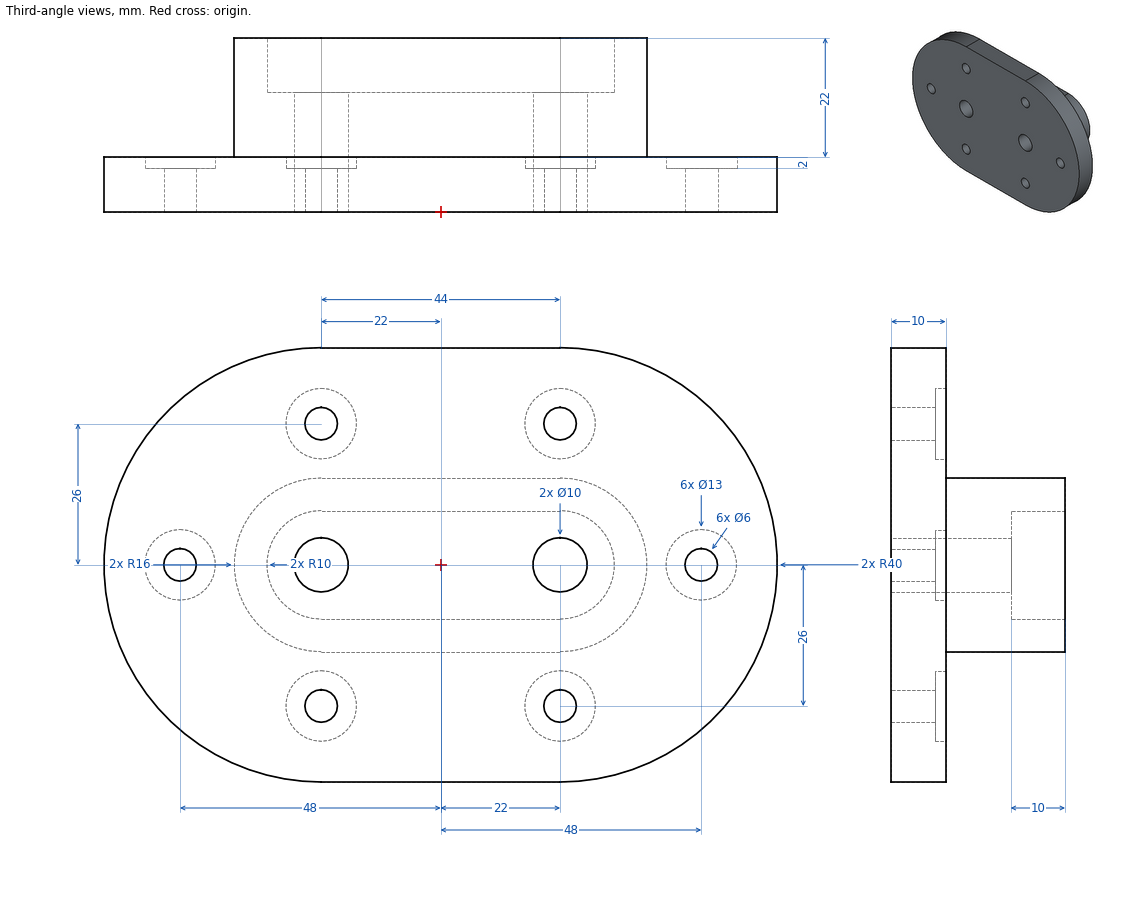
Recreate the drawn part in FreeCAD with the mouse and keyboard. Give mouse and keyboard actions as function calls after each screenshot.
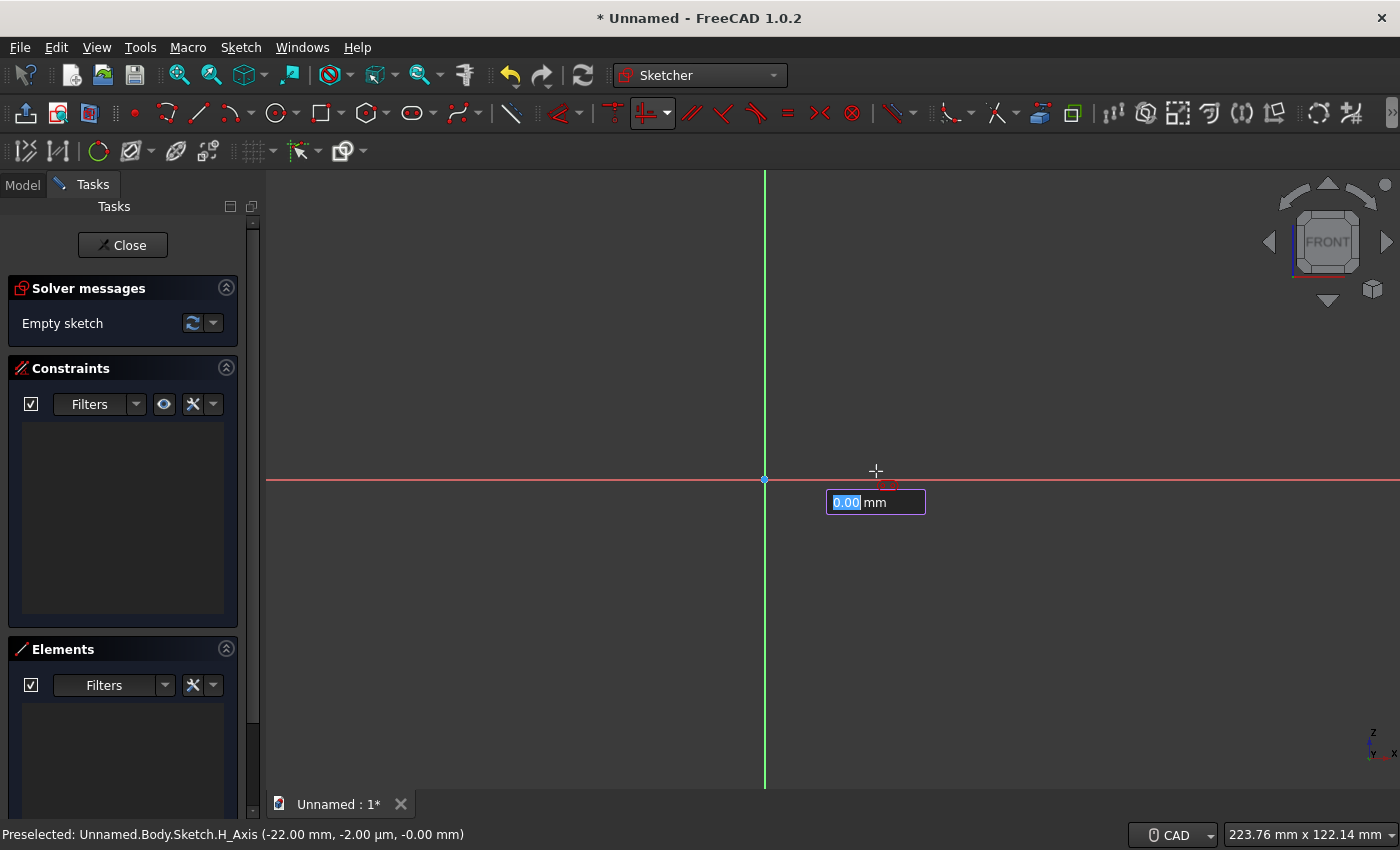
click(731, 277)
key(Escape)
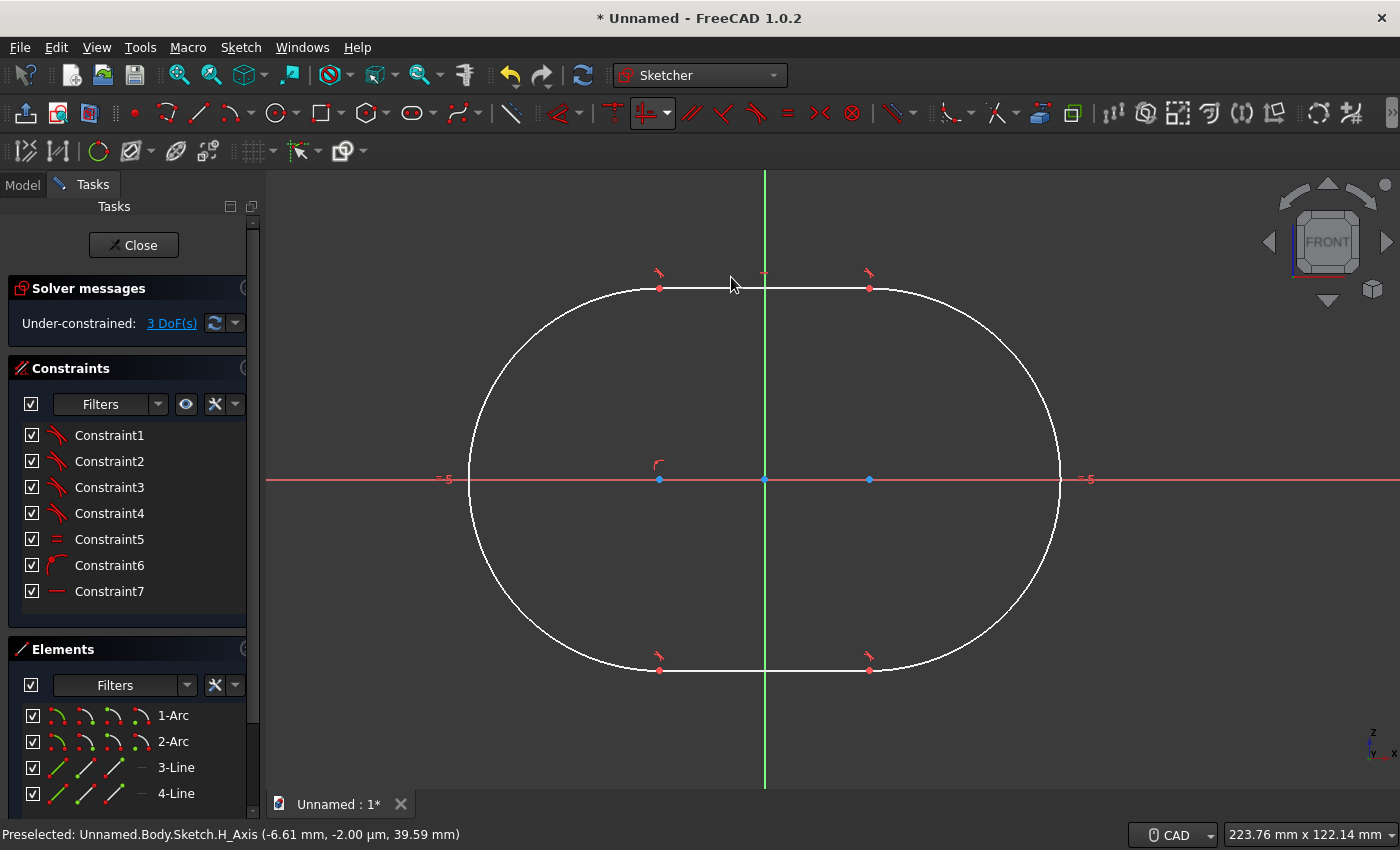
click(505, 367)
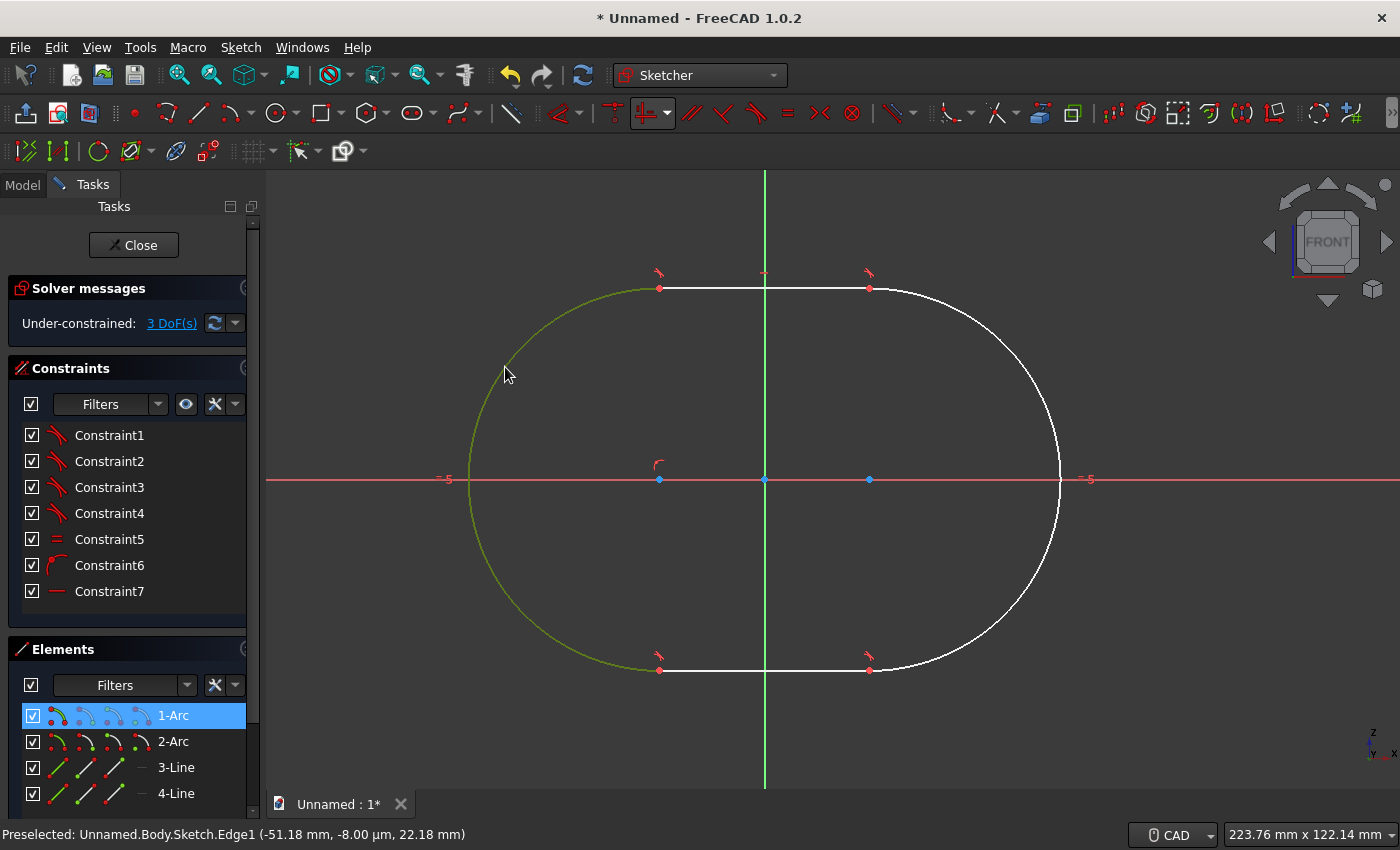
click(582, 114)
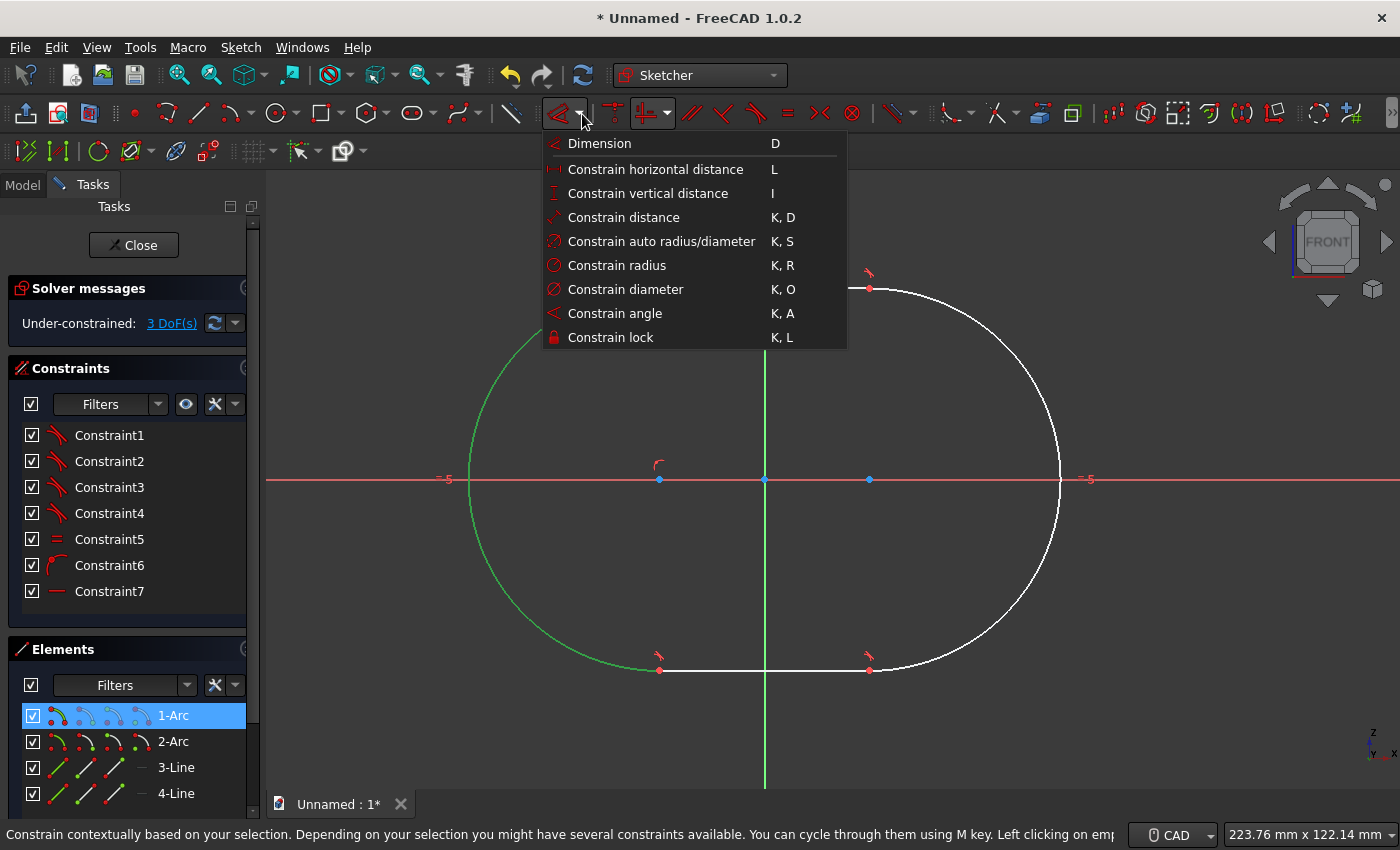
click(695, 265)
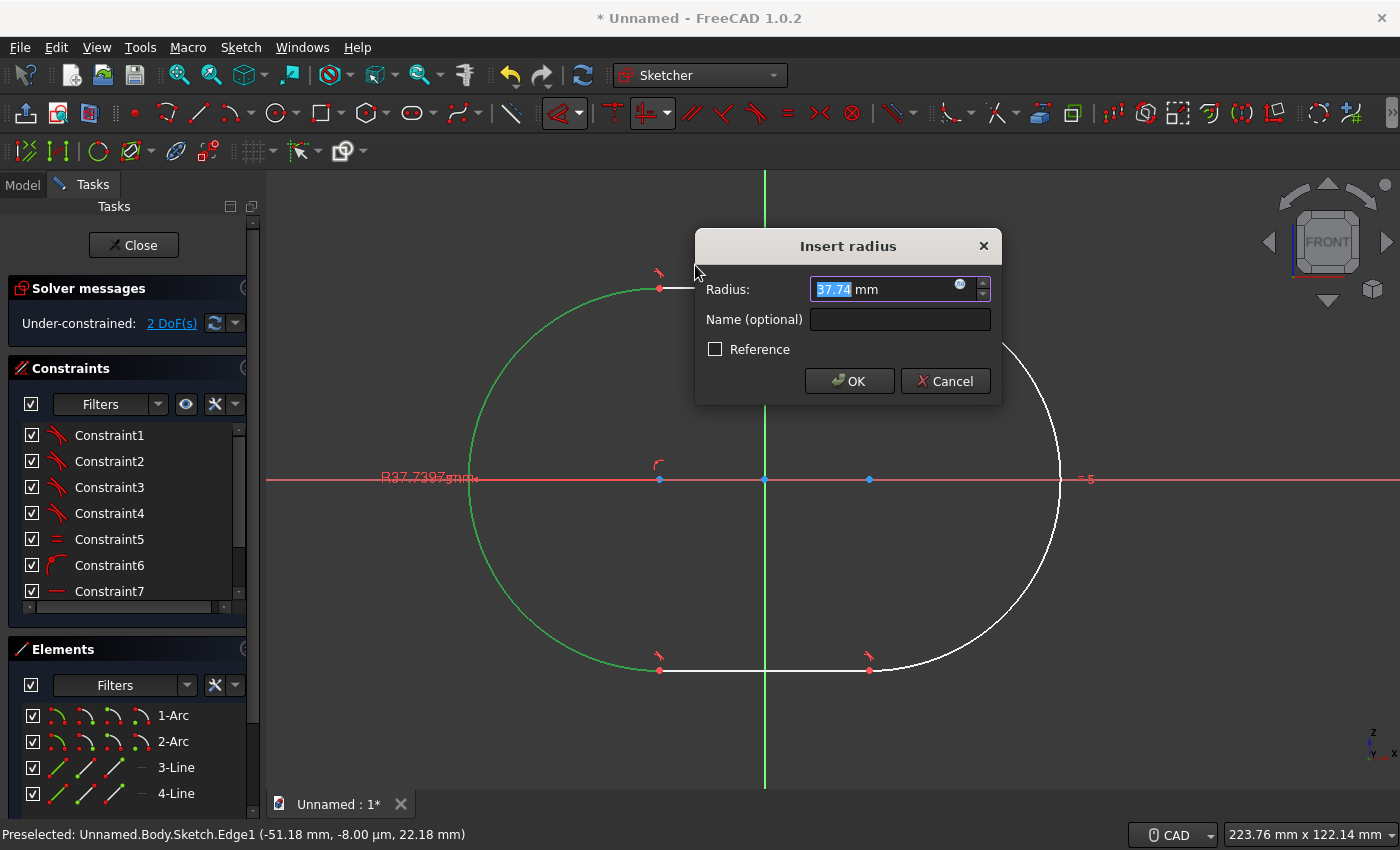
text(40)
key(Return)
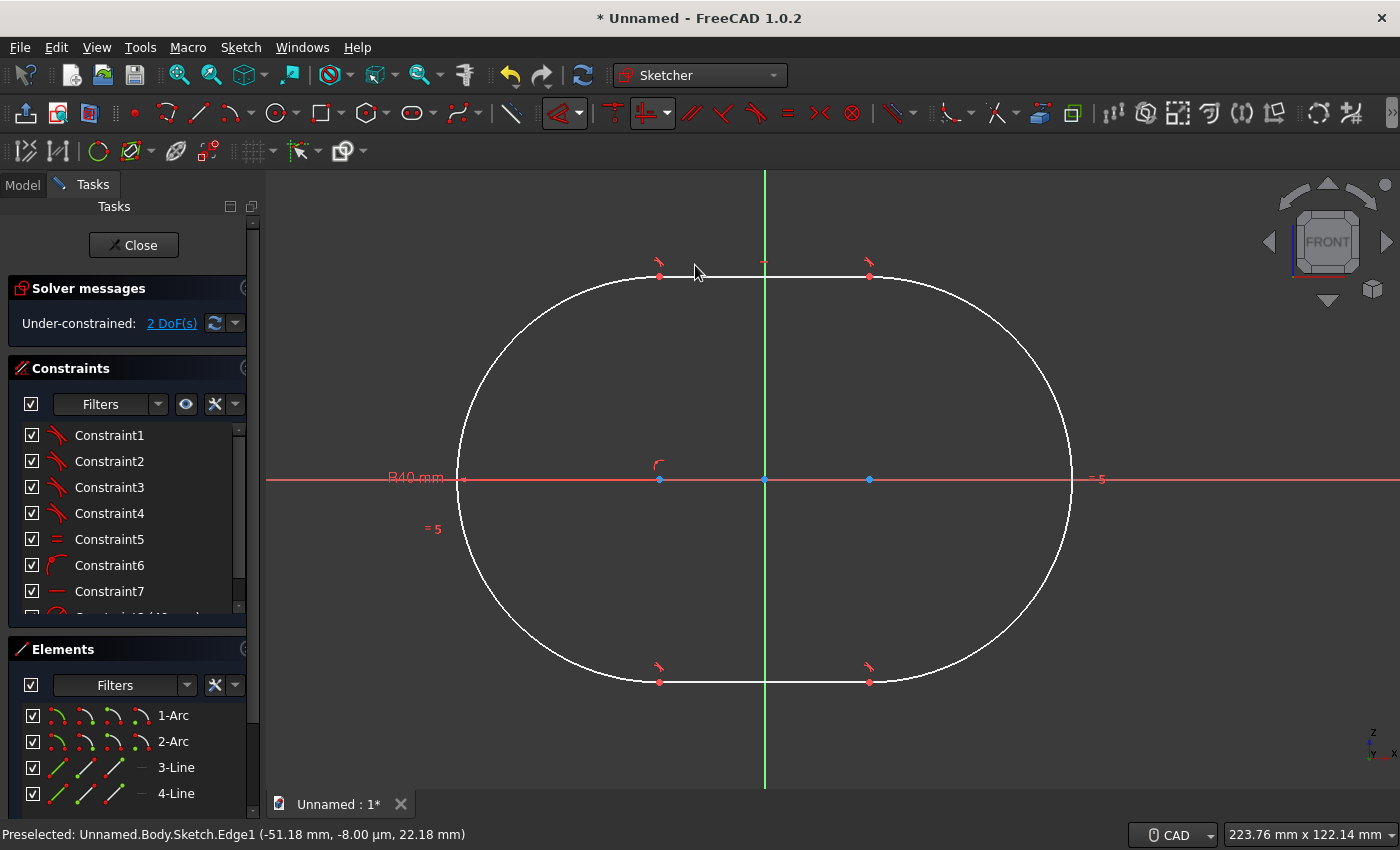
click(723, 277)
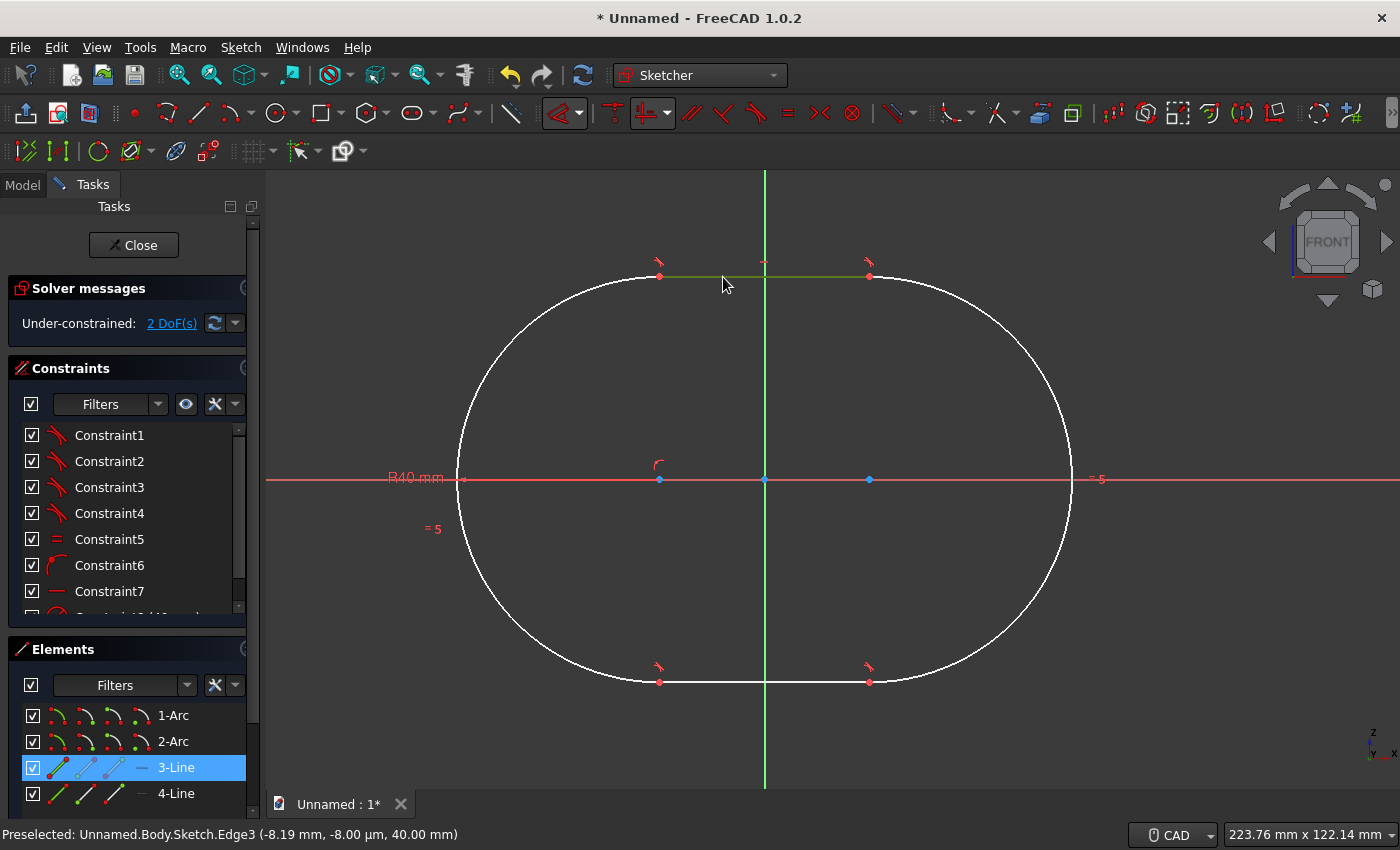
key(l)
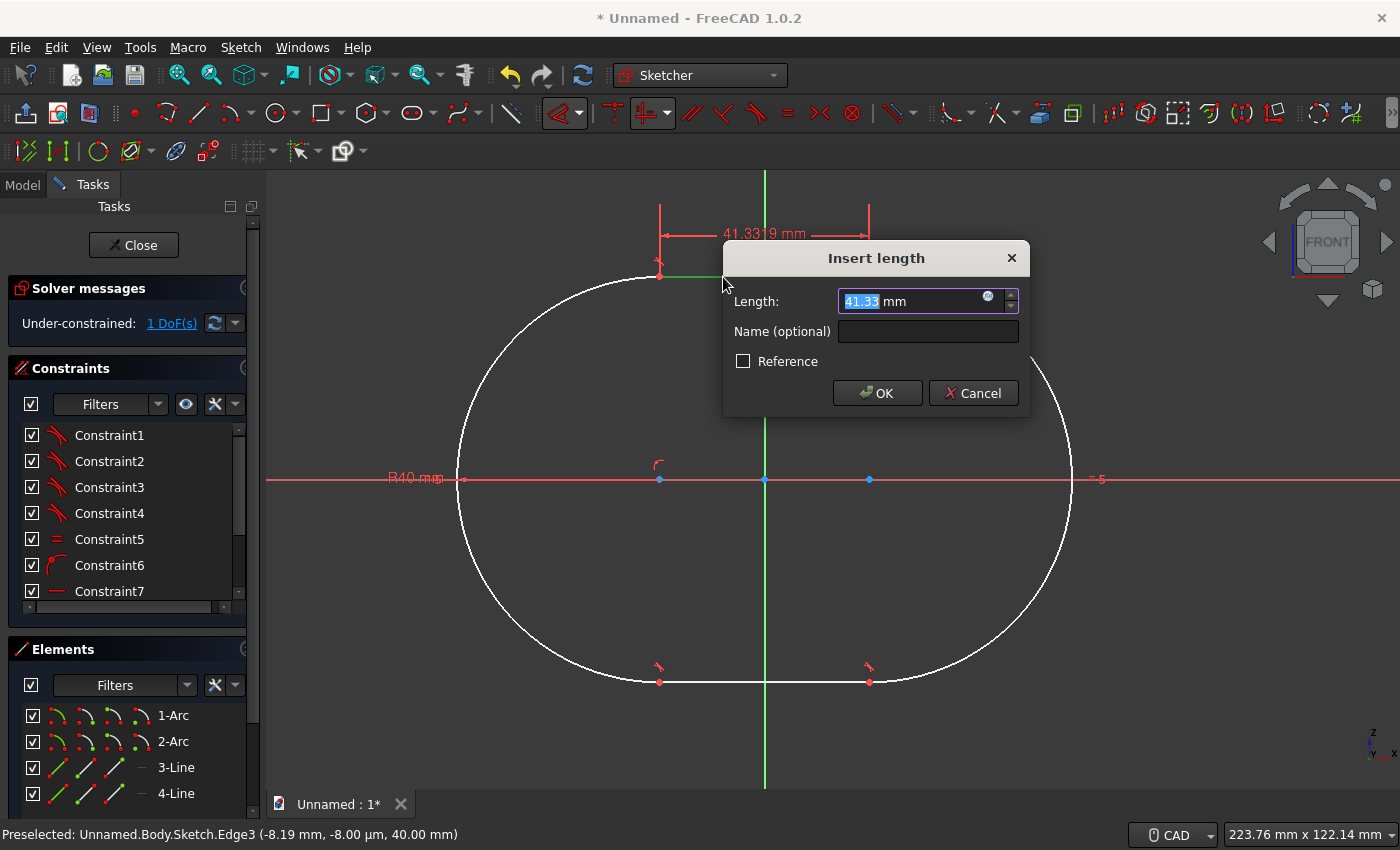
text(44)
key(Return)